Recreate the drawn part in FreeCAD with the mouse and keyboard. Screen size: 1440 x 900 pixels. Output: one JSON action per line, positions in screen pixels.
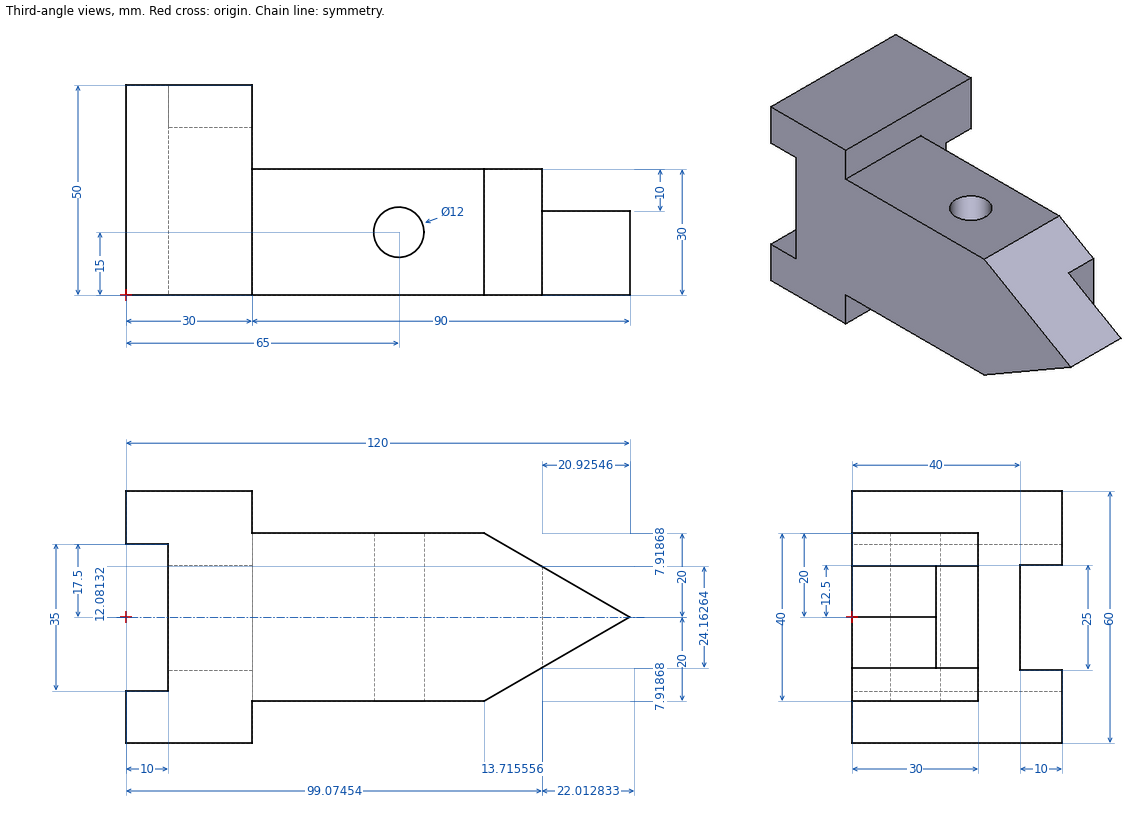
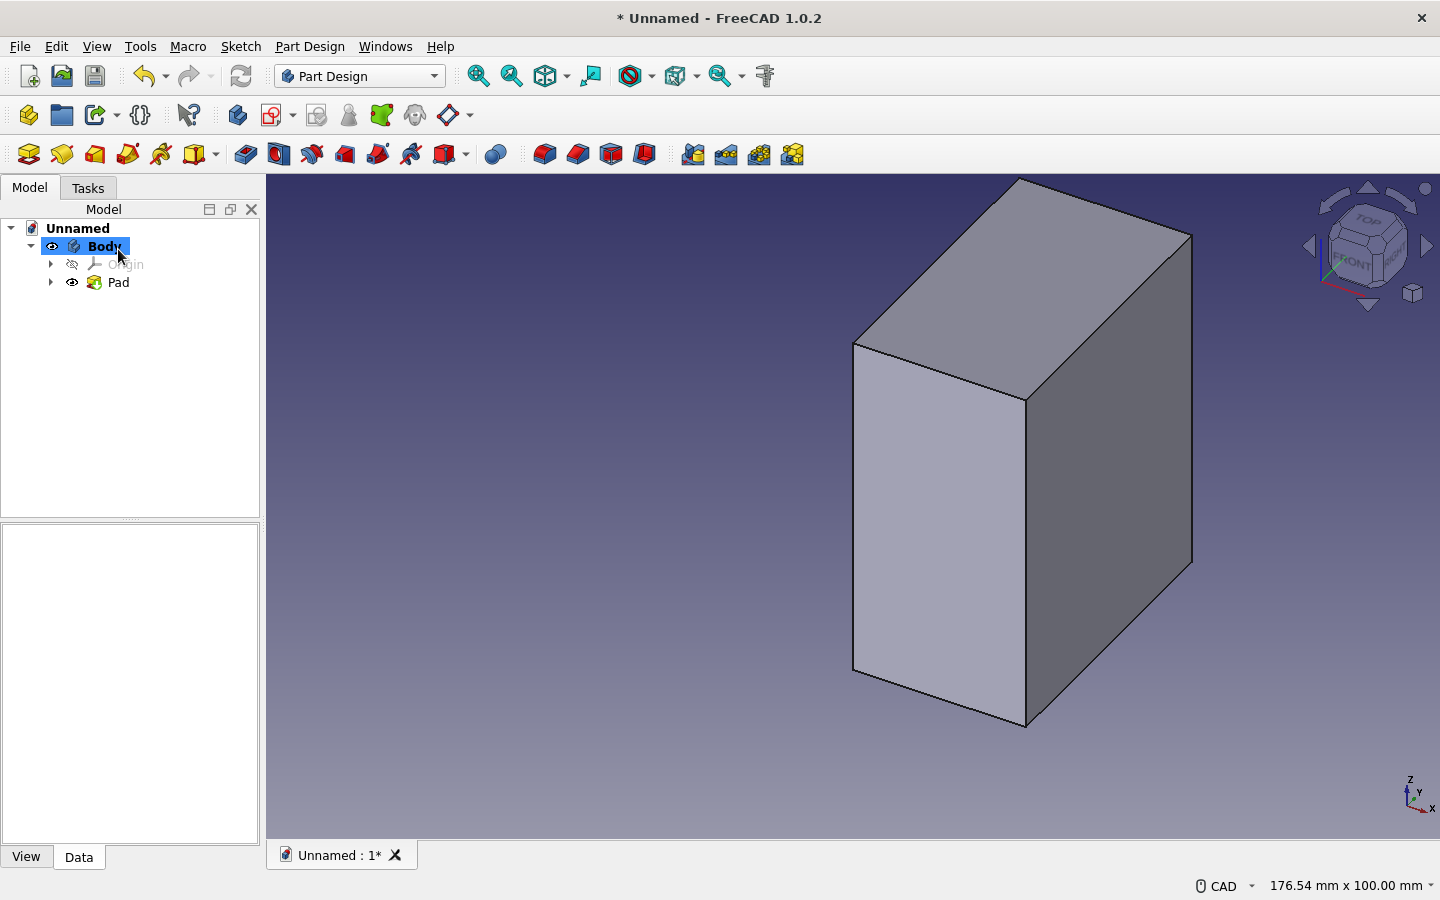
{"action": "key", "text": "4"}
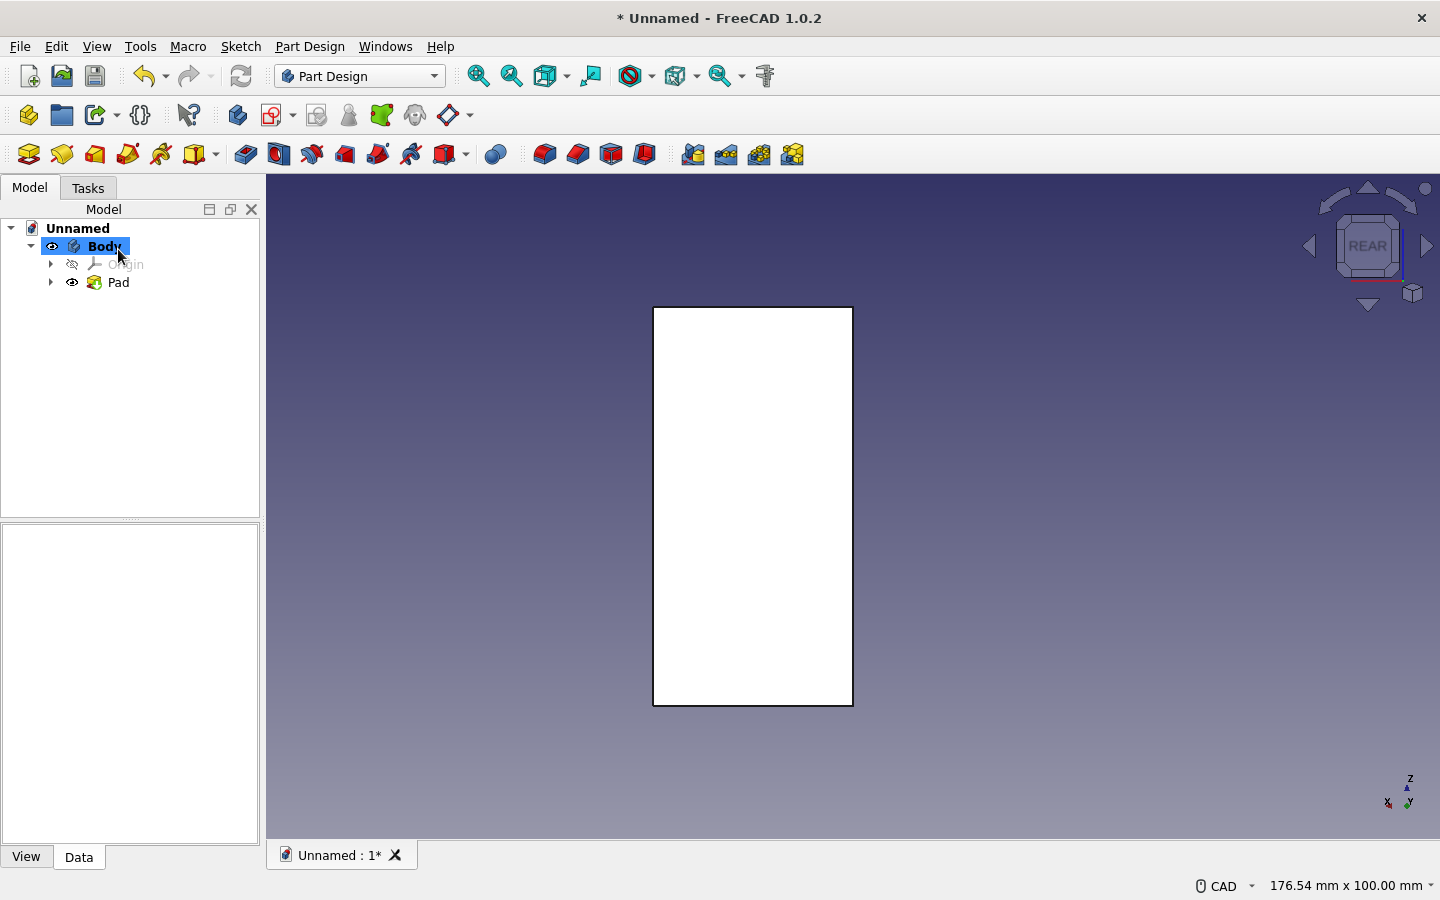
{"action": "left_click", "coordinate": [753, 448]}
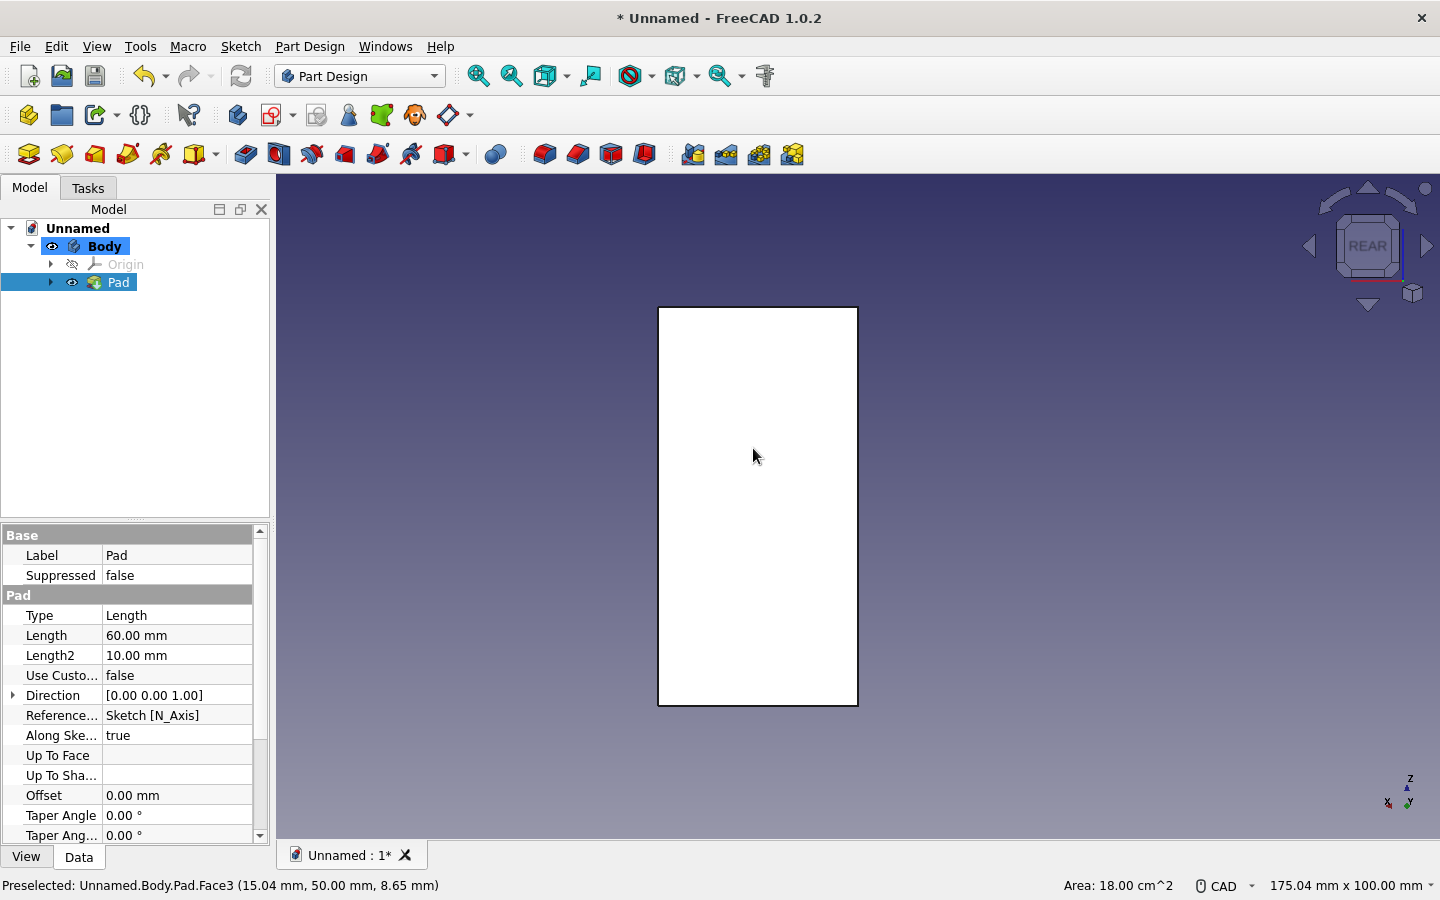
{"action": "left_click", "coordinate": [270, 116]}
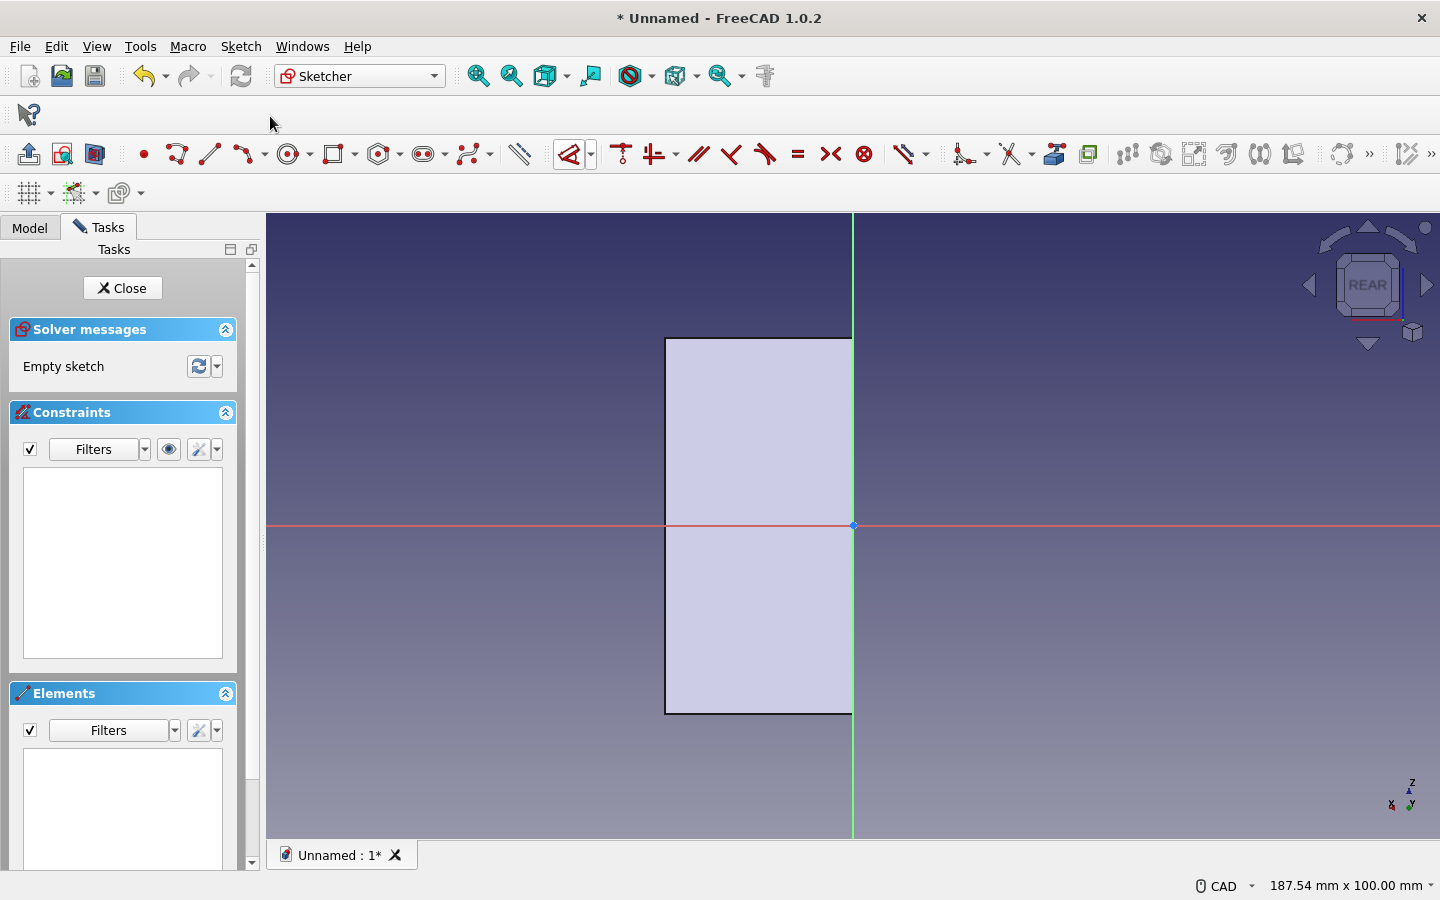
{"action": "scroll", "coordinate": [867, 526], "scroll_direction": "up", "scroll_amount": 3}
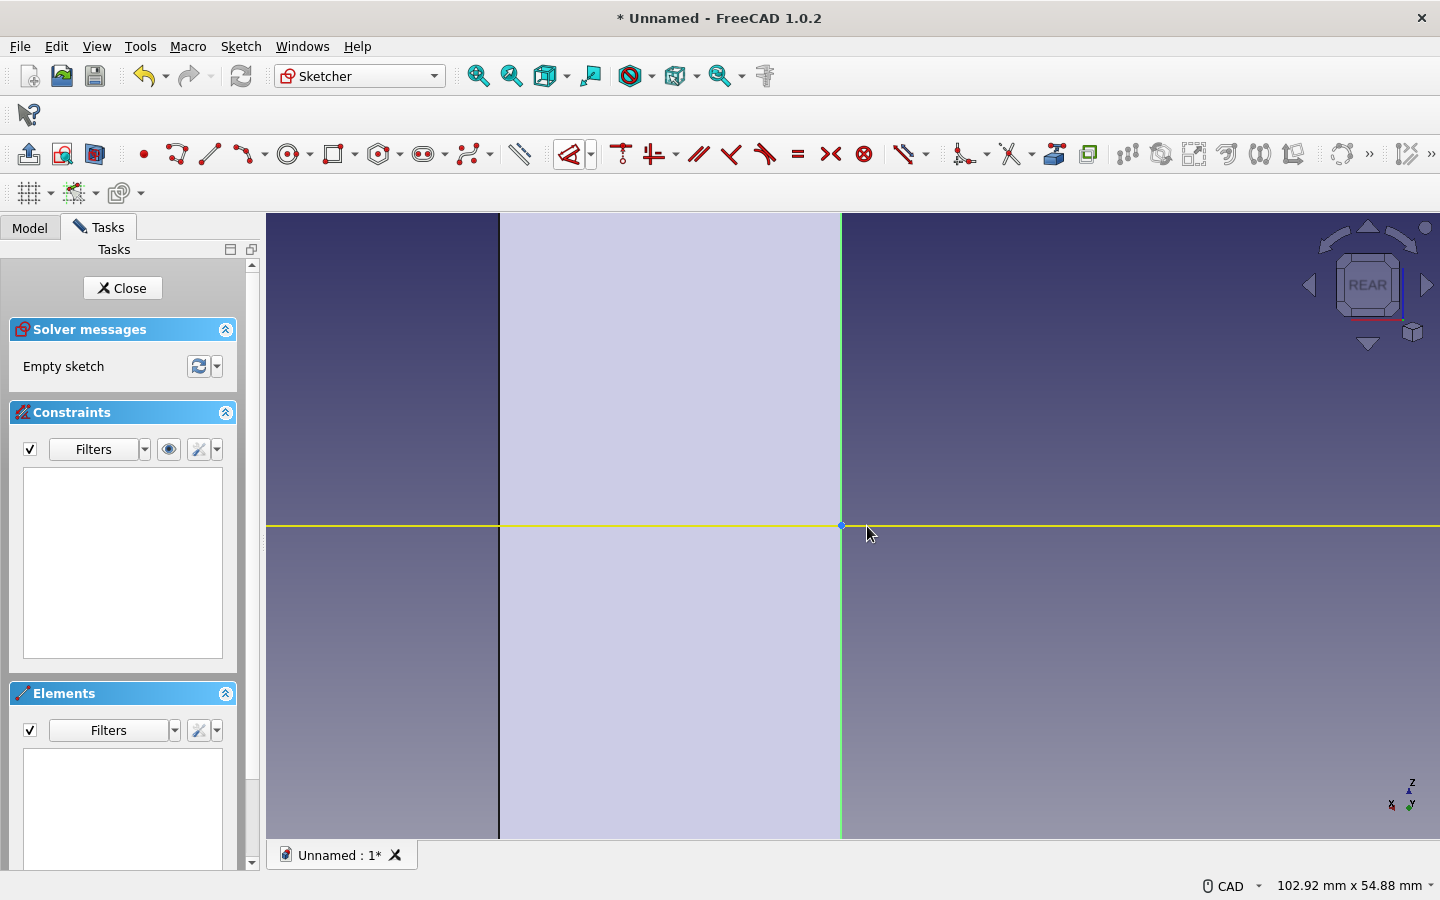
{"action": "left_click", "coordinate": [332, 154]}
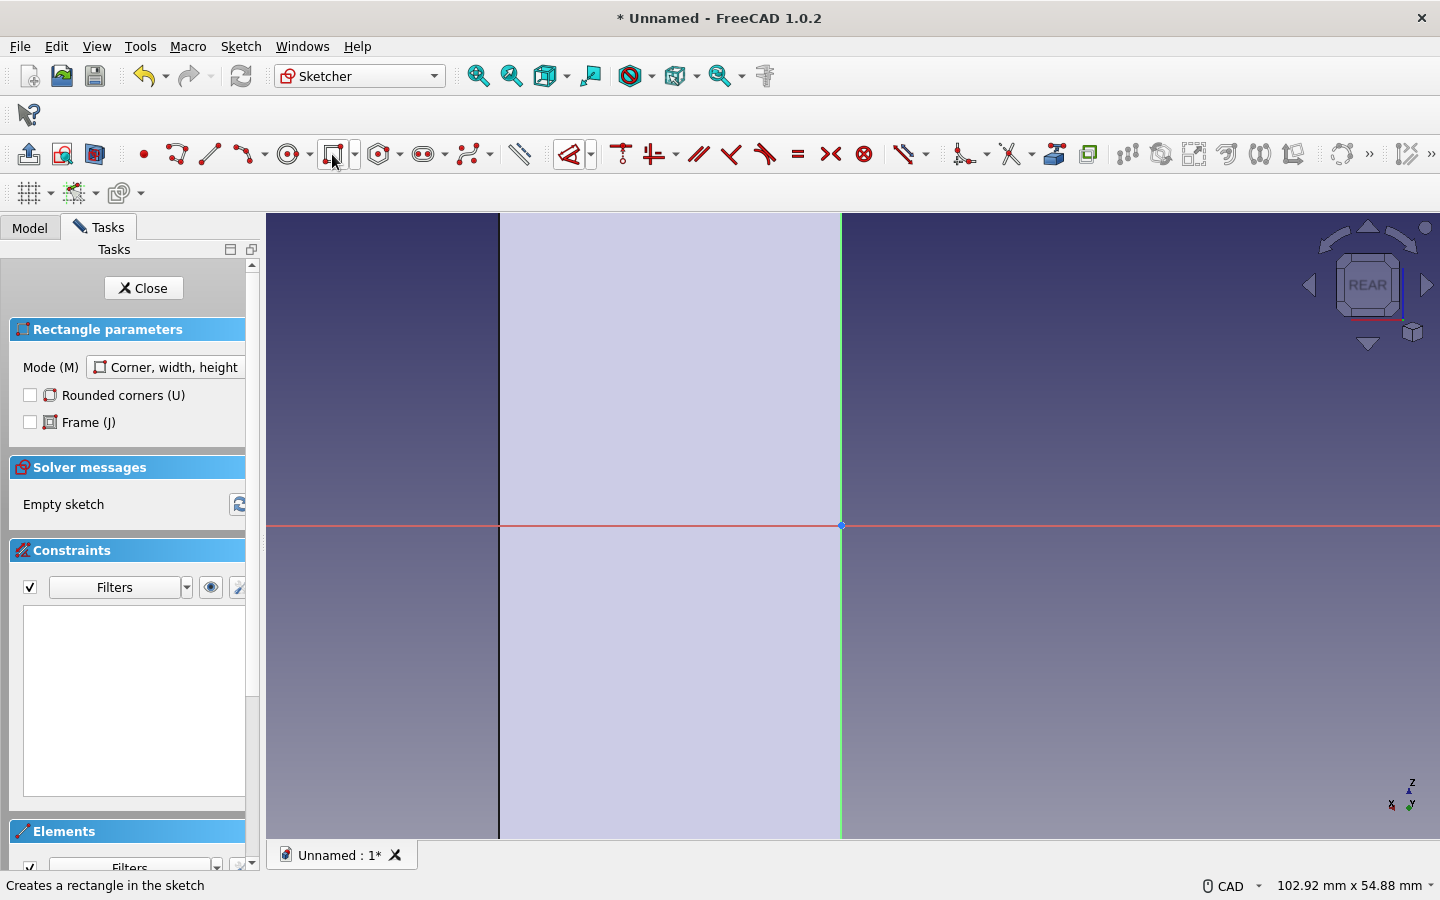
{"action": "left_click", "coordinate": [727, 326]}
{"action": "left_click", "coordinate": [841, 725]}
{"action": "key", "text": "Escape"}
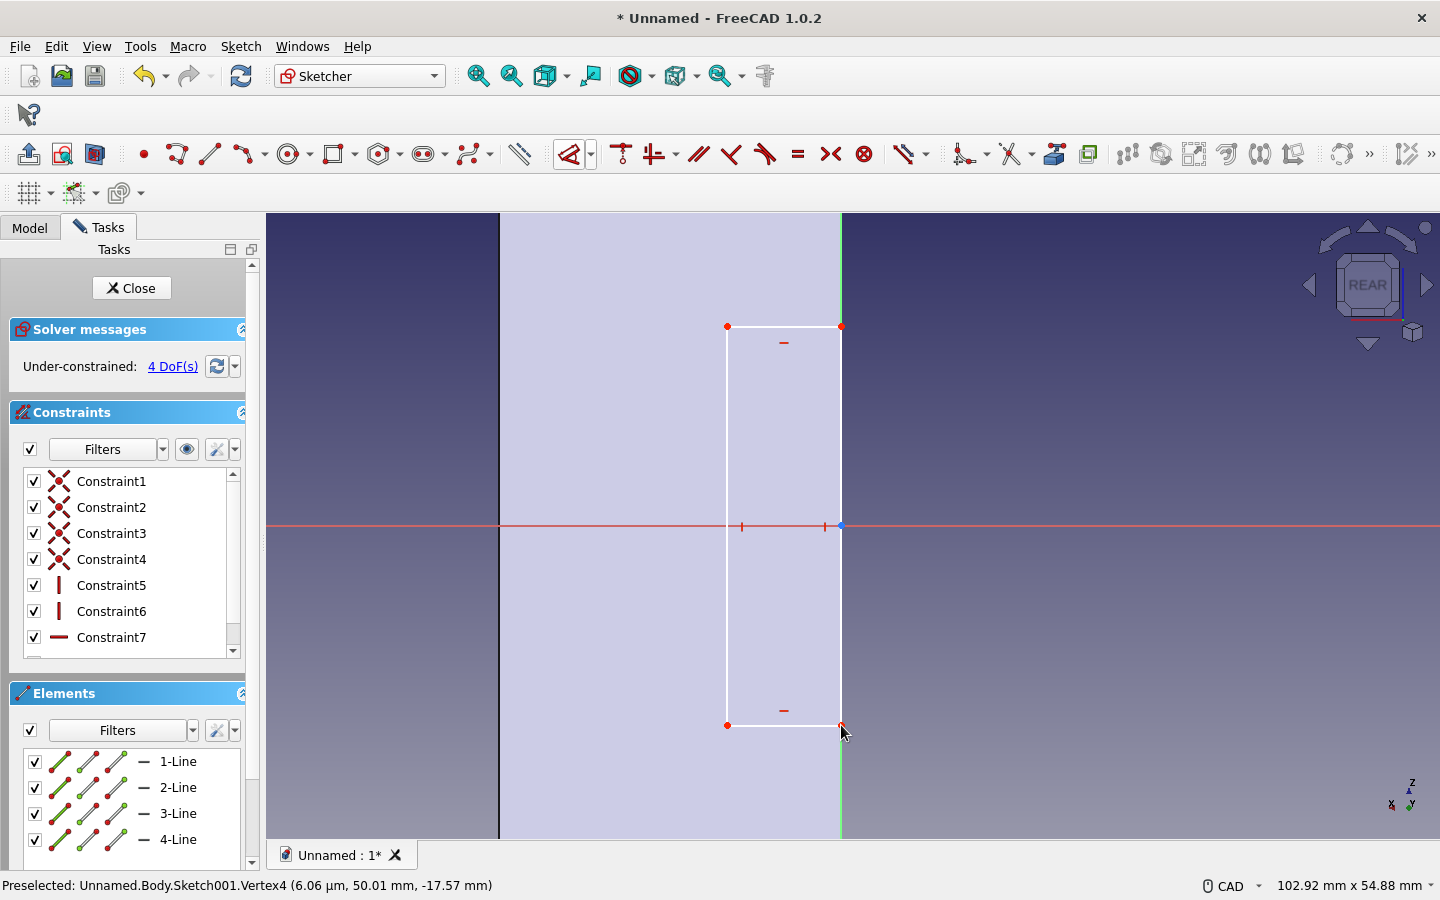
{"action": "left_click", "coordinate": [841, 726]}